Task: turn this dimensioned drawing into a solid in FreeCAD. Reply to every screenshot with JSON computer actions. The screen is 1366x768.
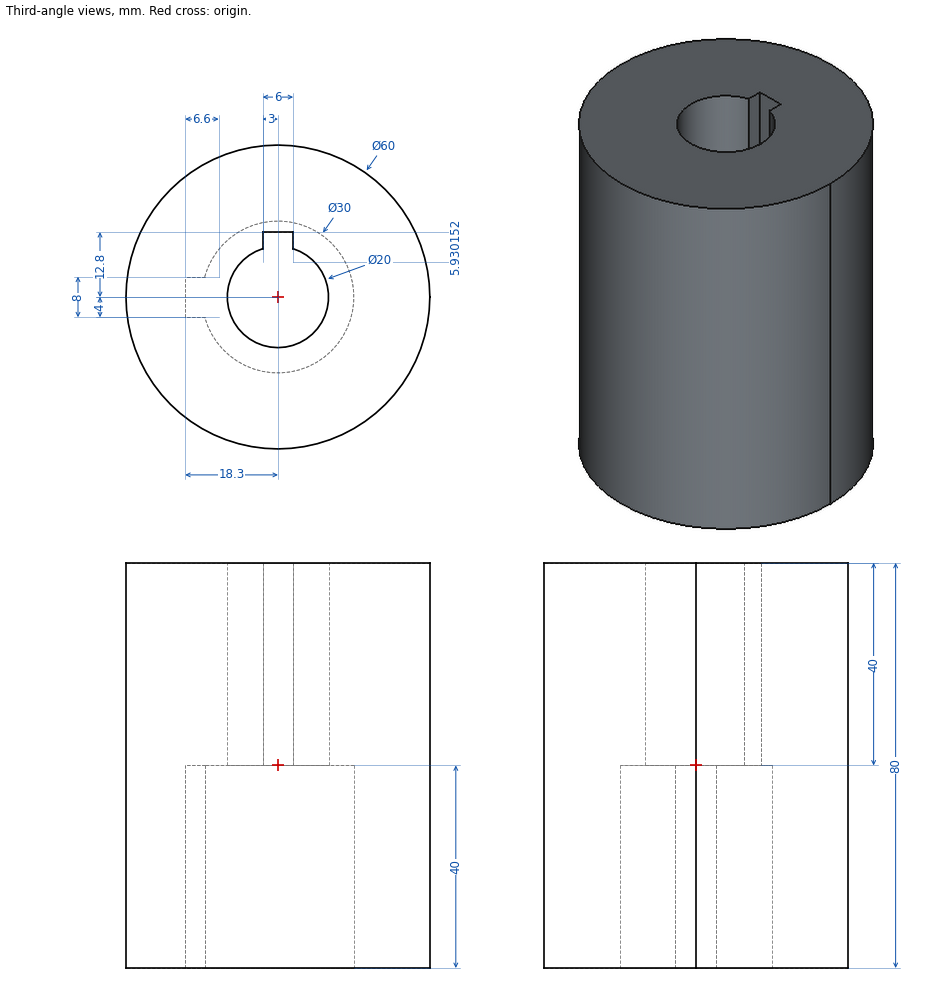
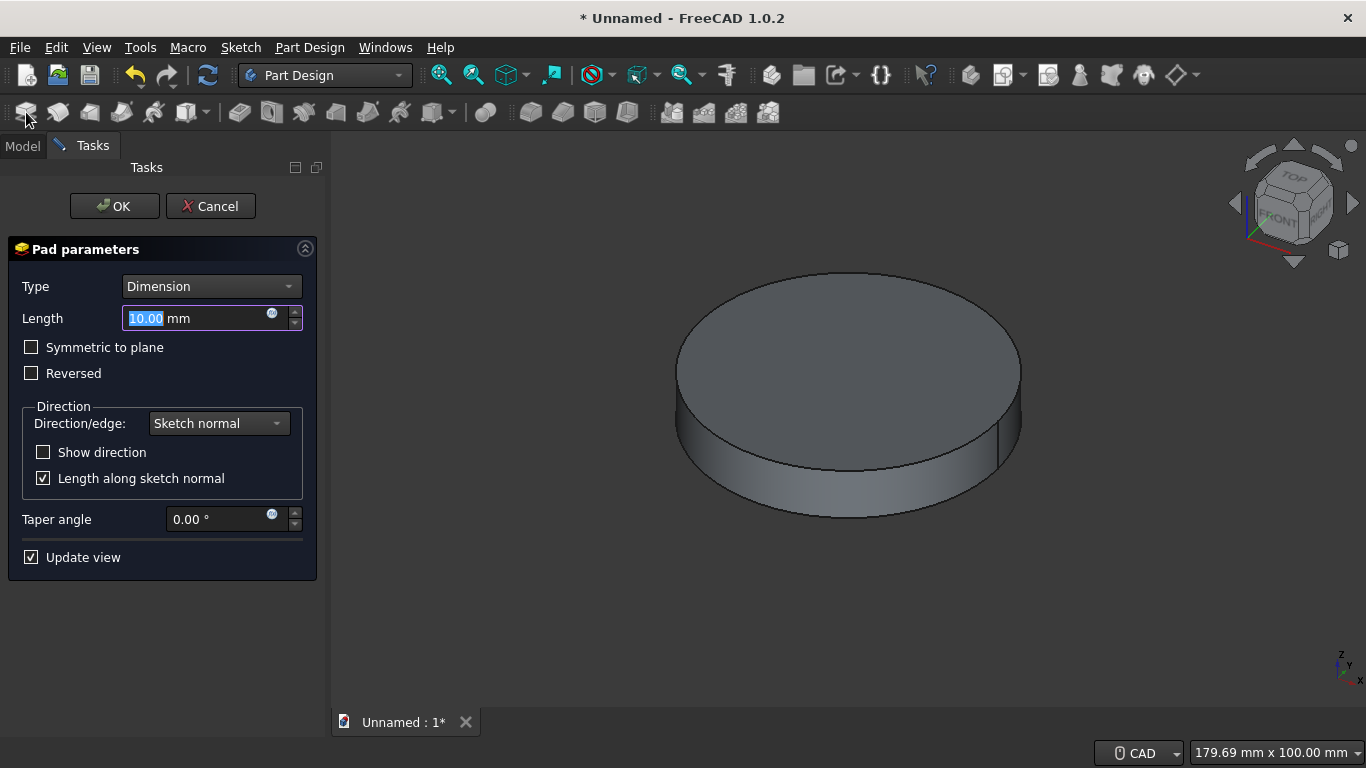
{"action": "type", "text": "80"}
{"action": "key", "text": "Tab"}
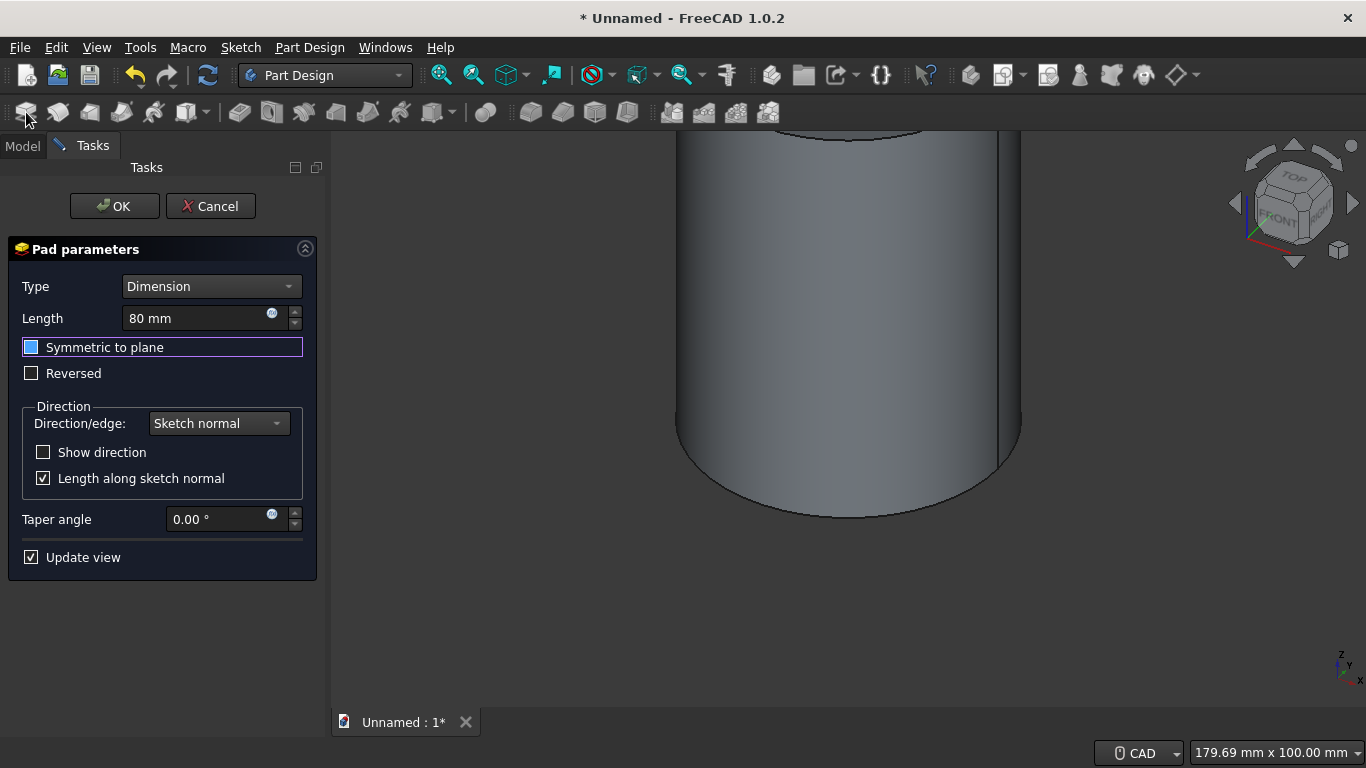
{"action": "left_click", "coordinate": [30, 347]}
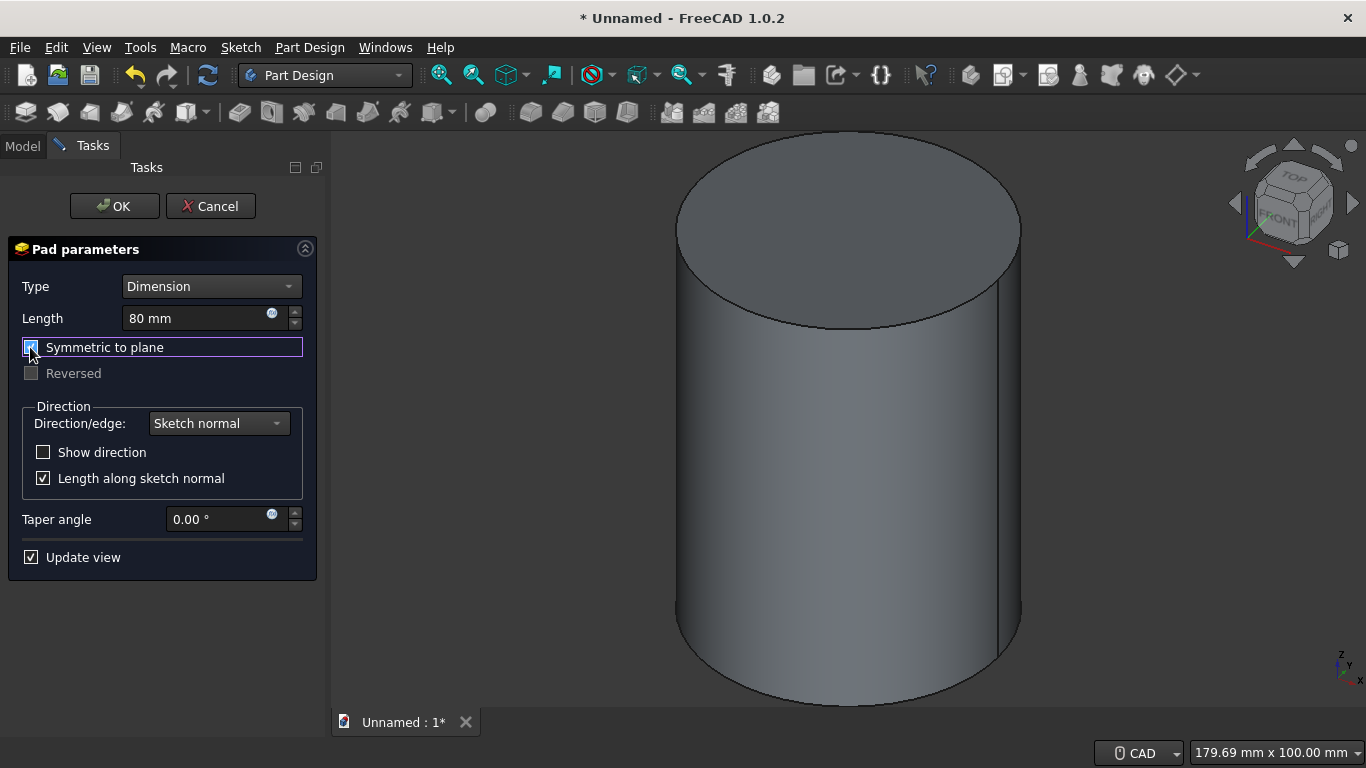
{"action": "left_click", "coordinate": [115, 206]}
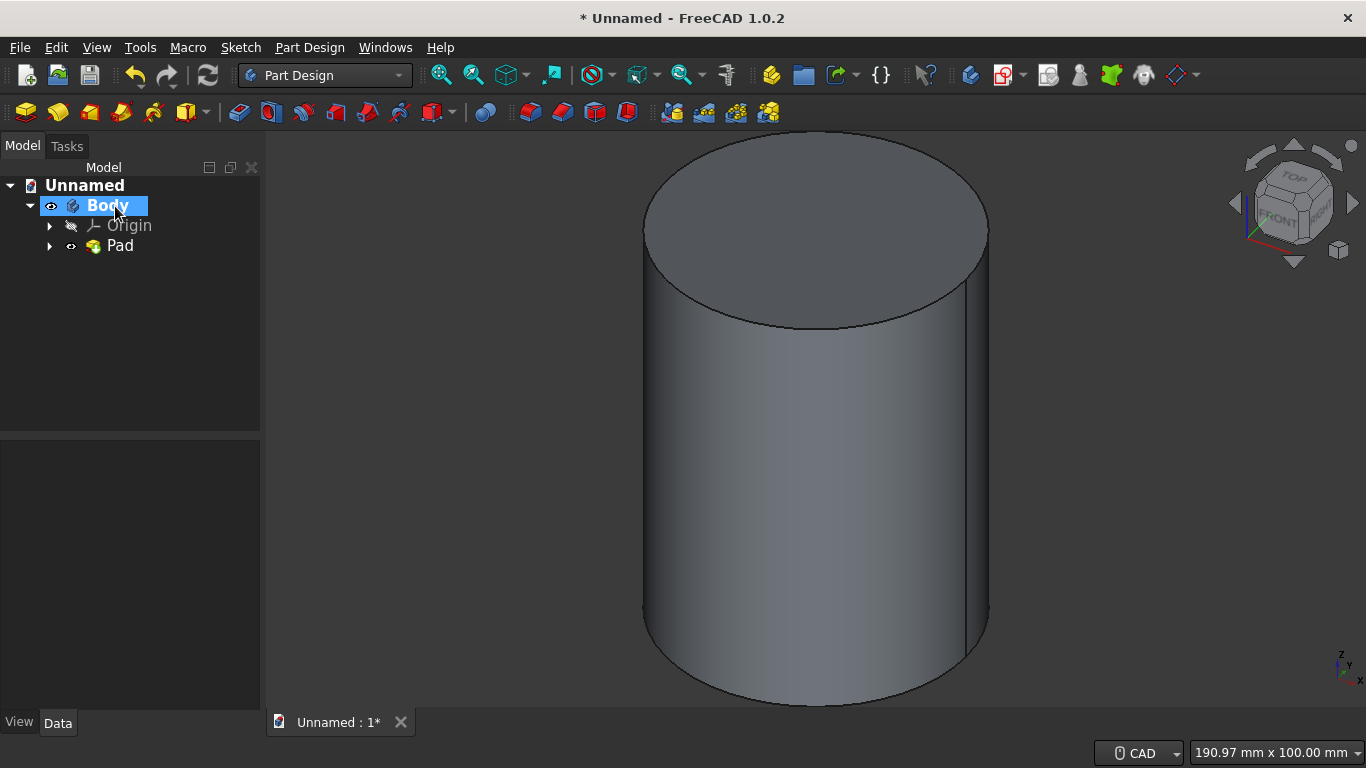
{"action": "key", "text": "v f"}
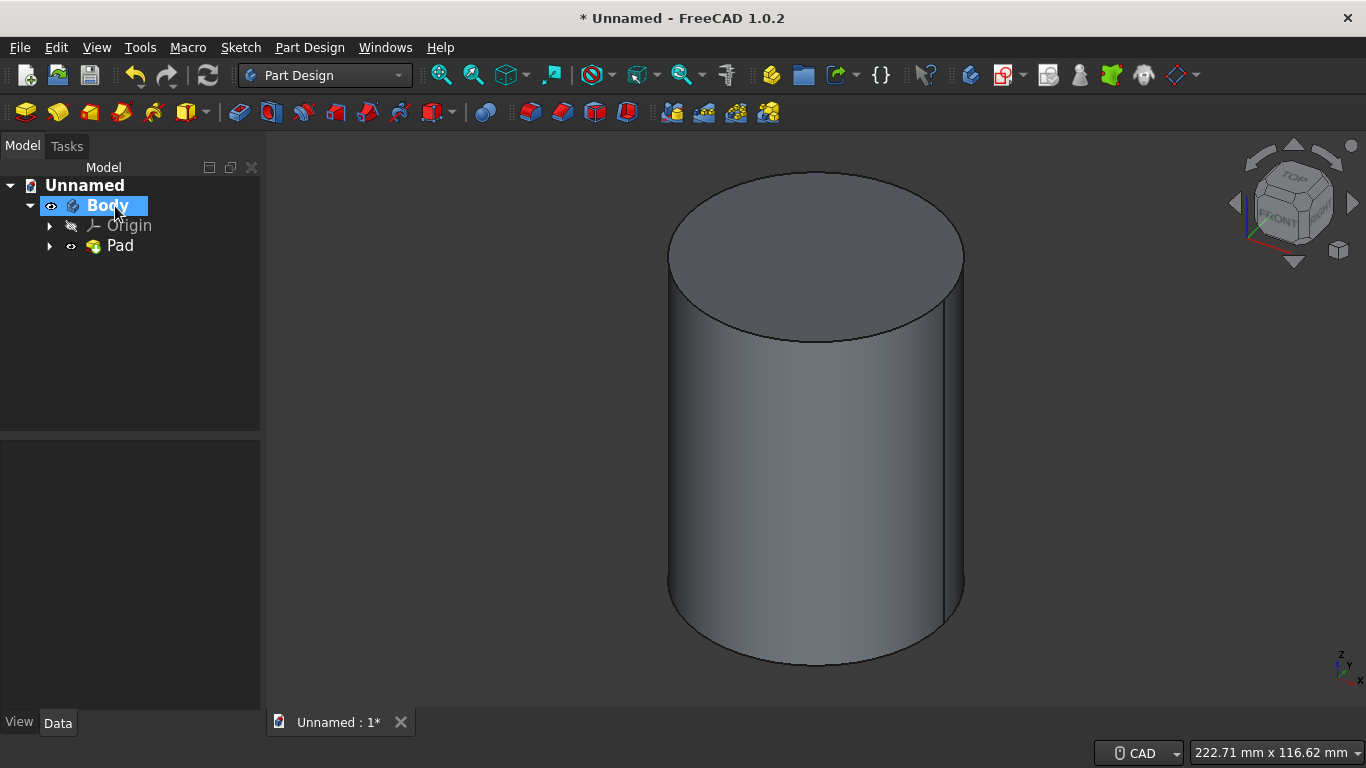
{"action": "left_click", "coordinate": [816, 256]}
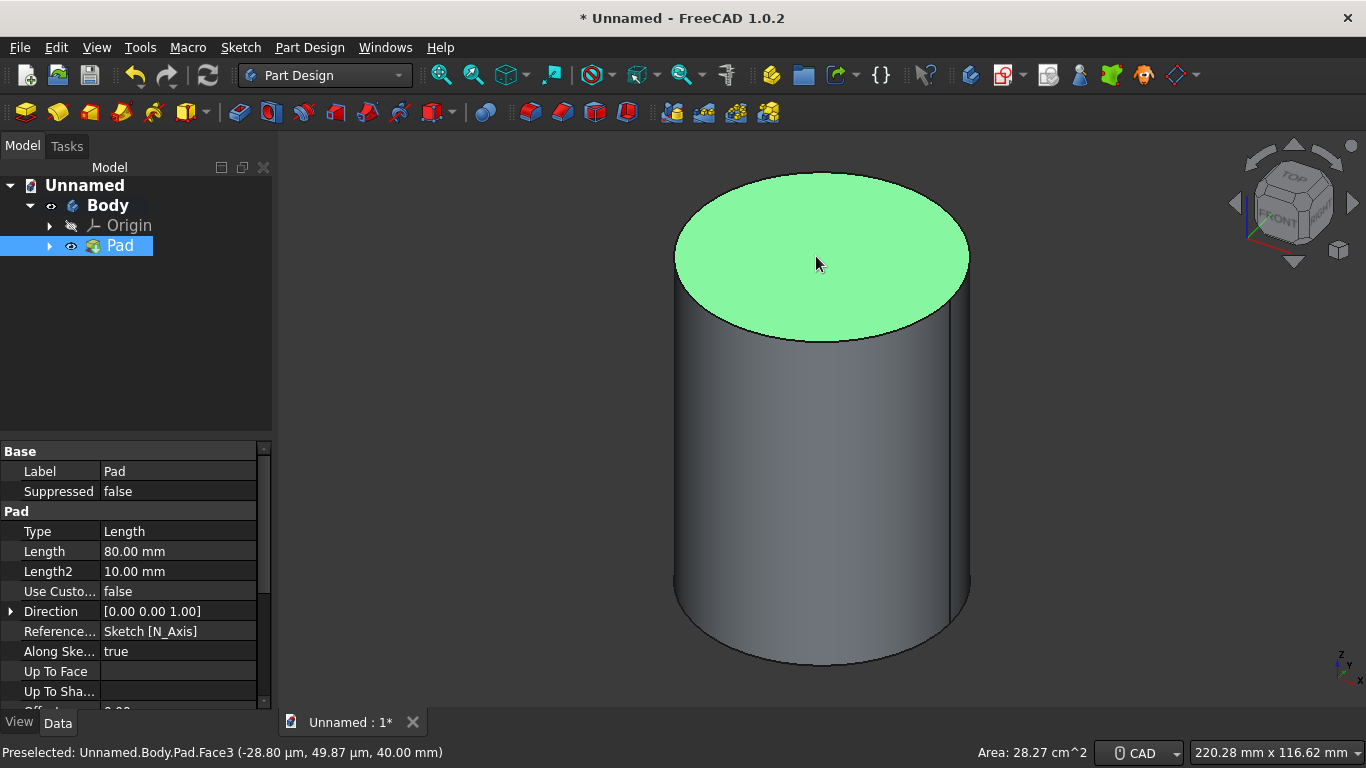
{"action": "left_click", "coordinate": [1004, 76]}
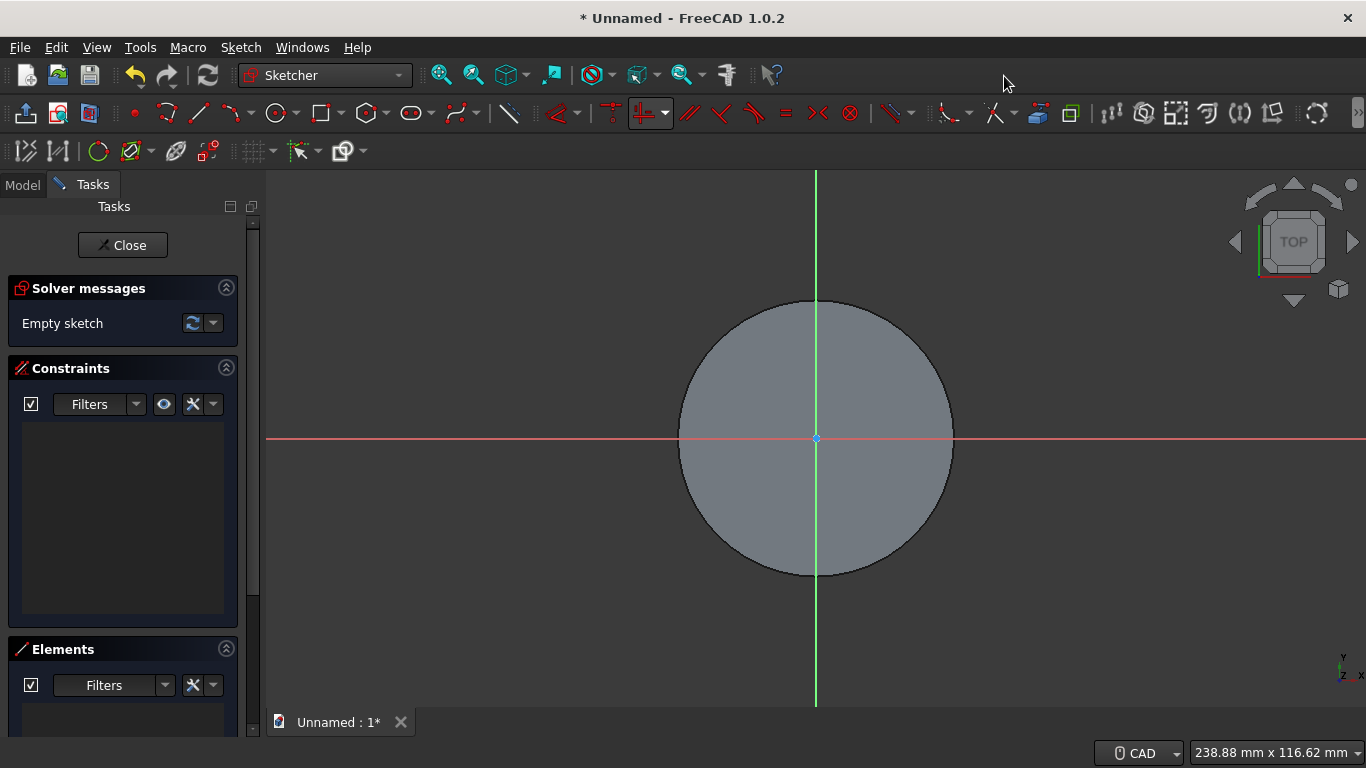
{"action": "scroll", "coordinate": [838, 438], "scroll_direction": "up", "scroll_amount": 7}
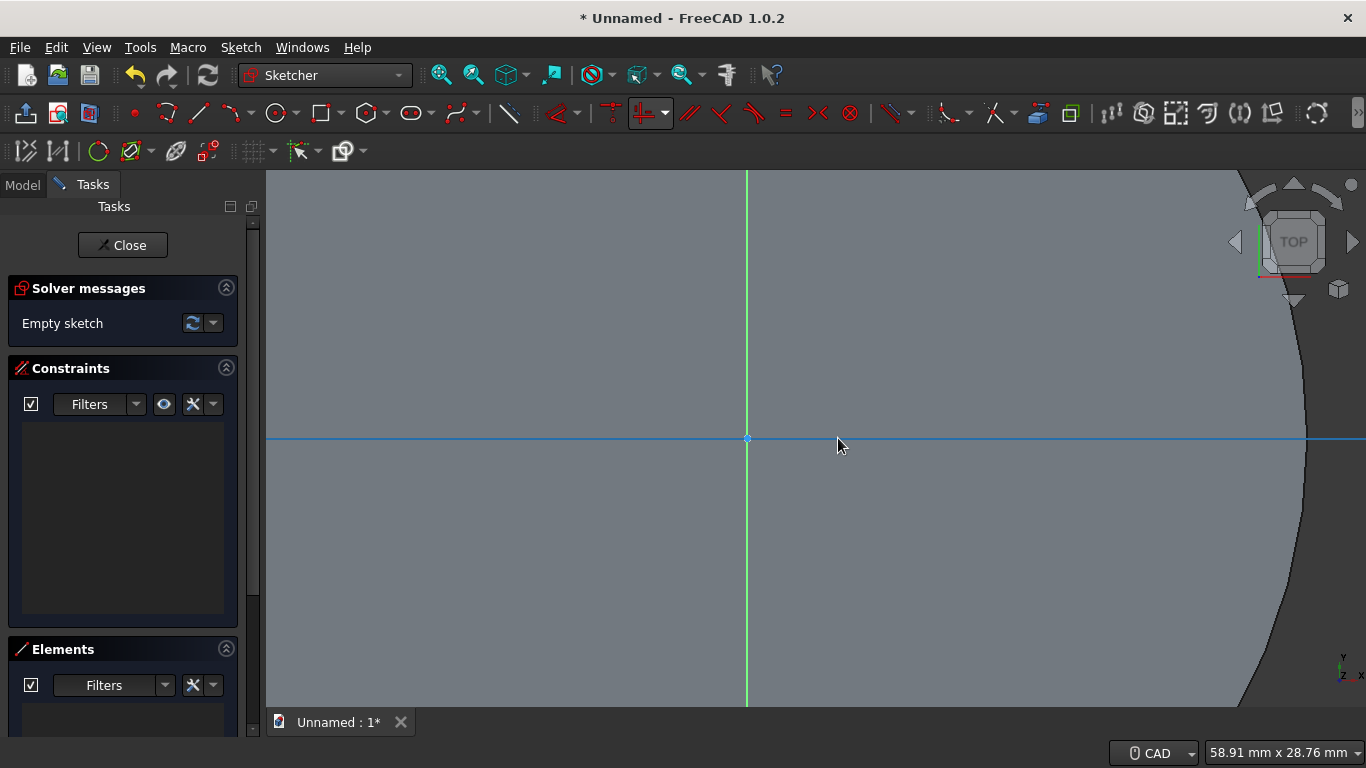
{"action": "key", "text": "g c"}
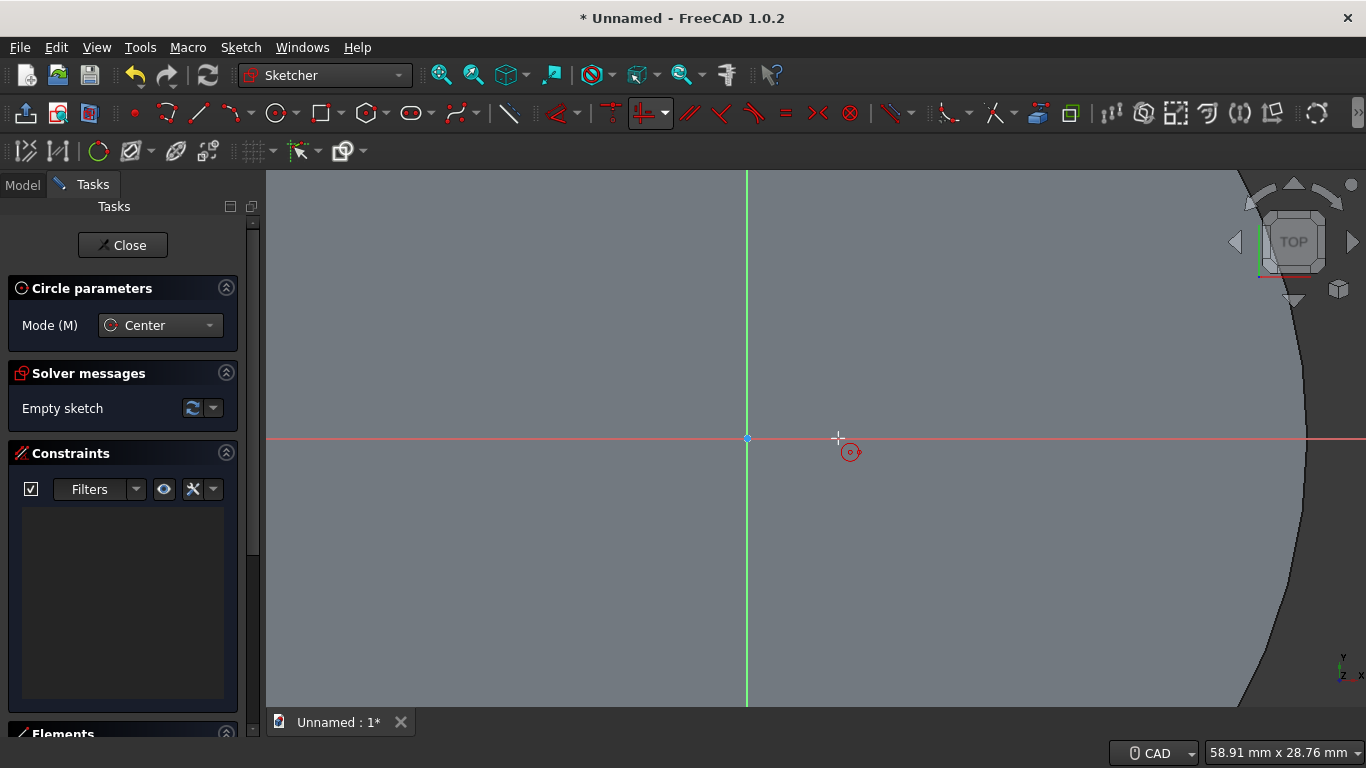
{"action": "left_click", "coordinate": [747, 438]}
{"action": "mouse_move", "coordinate": [879, 306]}